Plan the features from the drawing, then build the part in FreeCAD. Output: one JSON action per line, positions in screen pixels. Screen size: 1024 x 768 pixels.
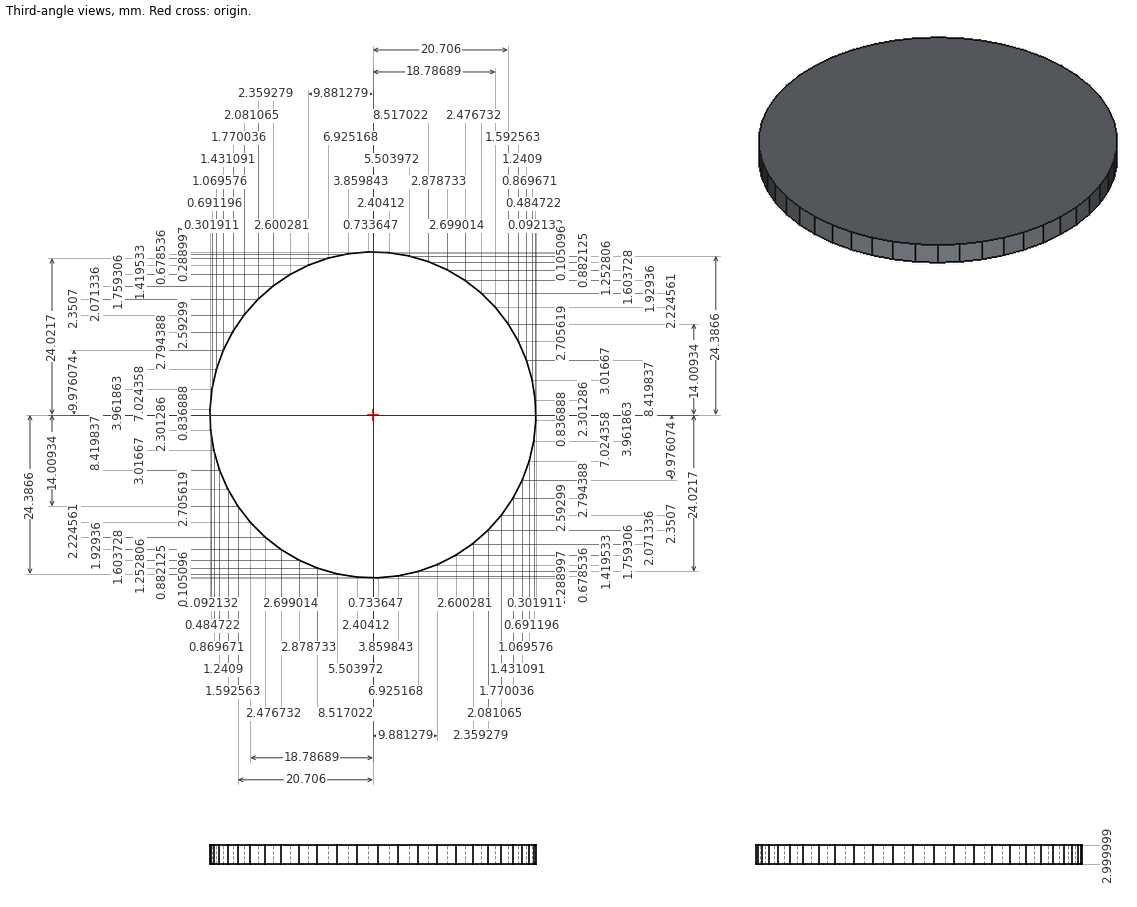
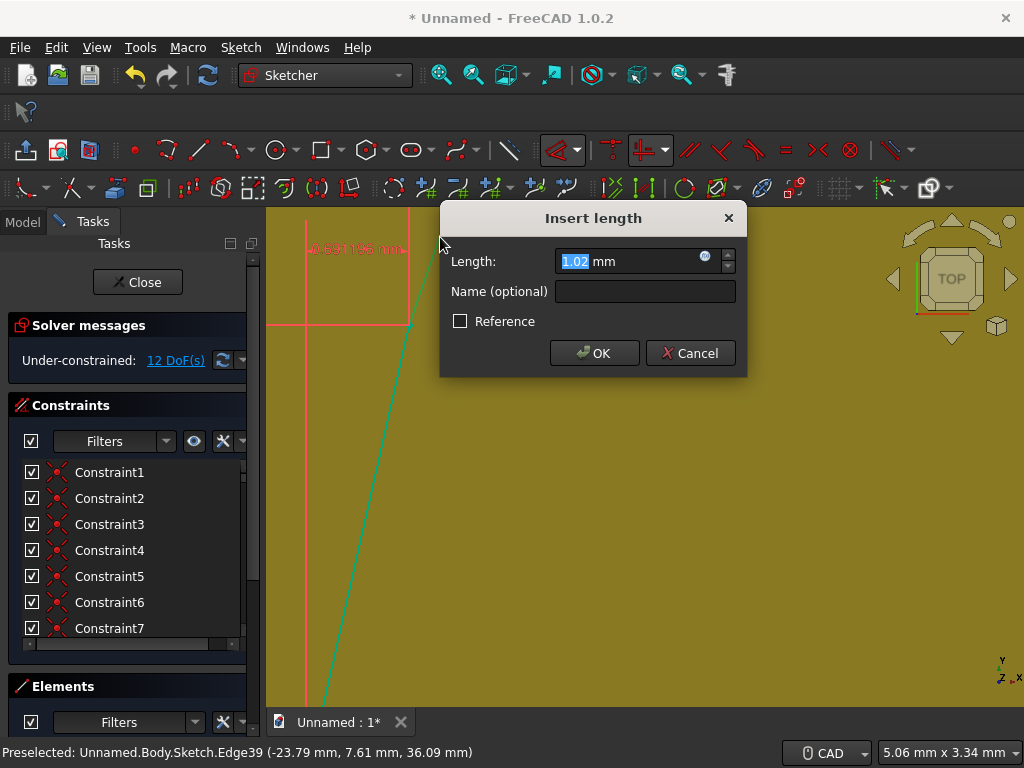
{"action": "type", "text": "1.069576"}
{"action": "key", "text": "Return"}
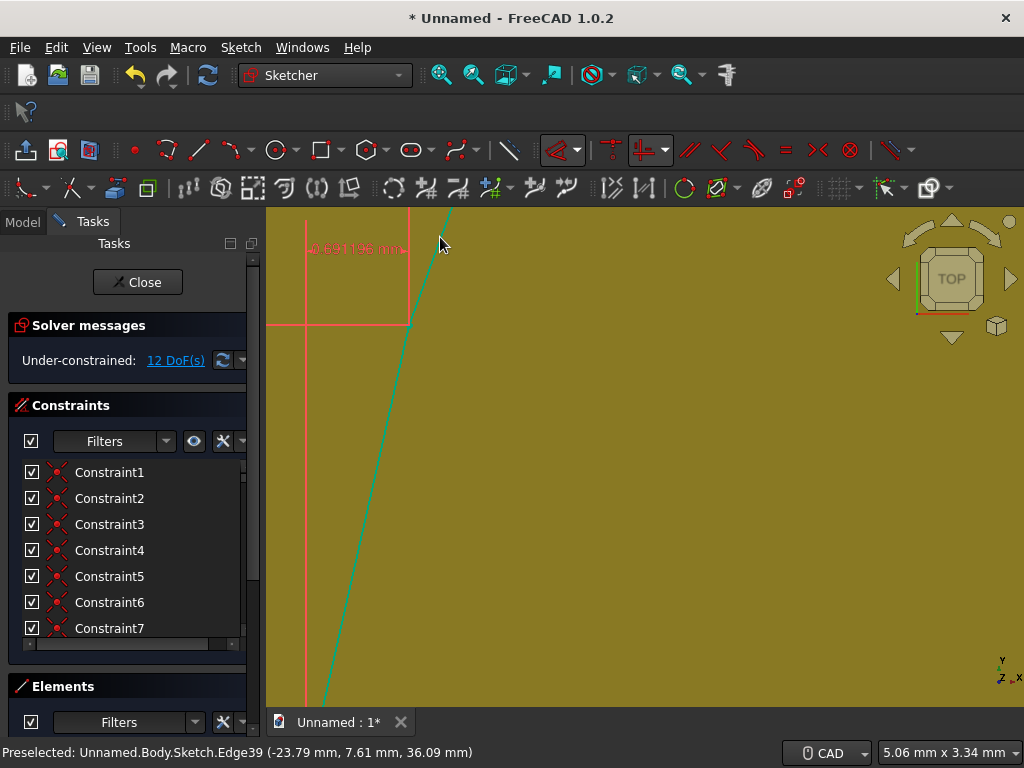
{"action": "scroll", "coordinate": [397, 409], "scroll_direction": "down", "scroll_amount": 15}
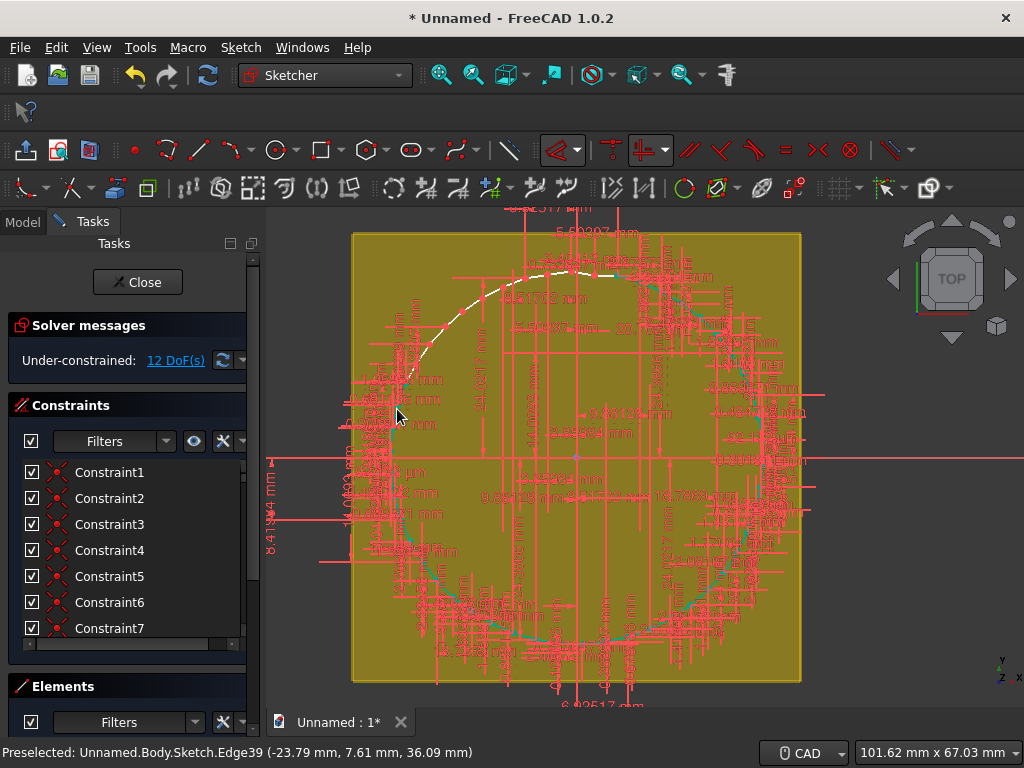
{"action": "scroll", "coordinate": [409, 377], "scroll_direction": "up", "scroll_amount": 7}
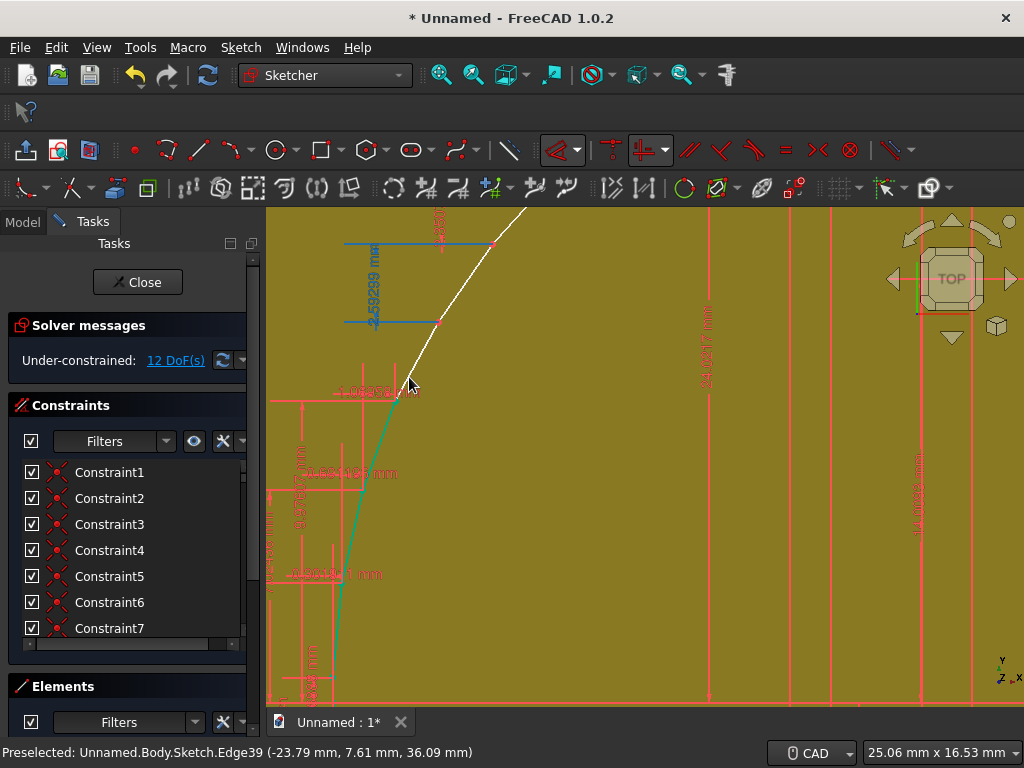
{"action": "left_click", "coordinate": [408, 378]}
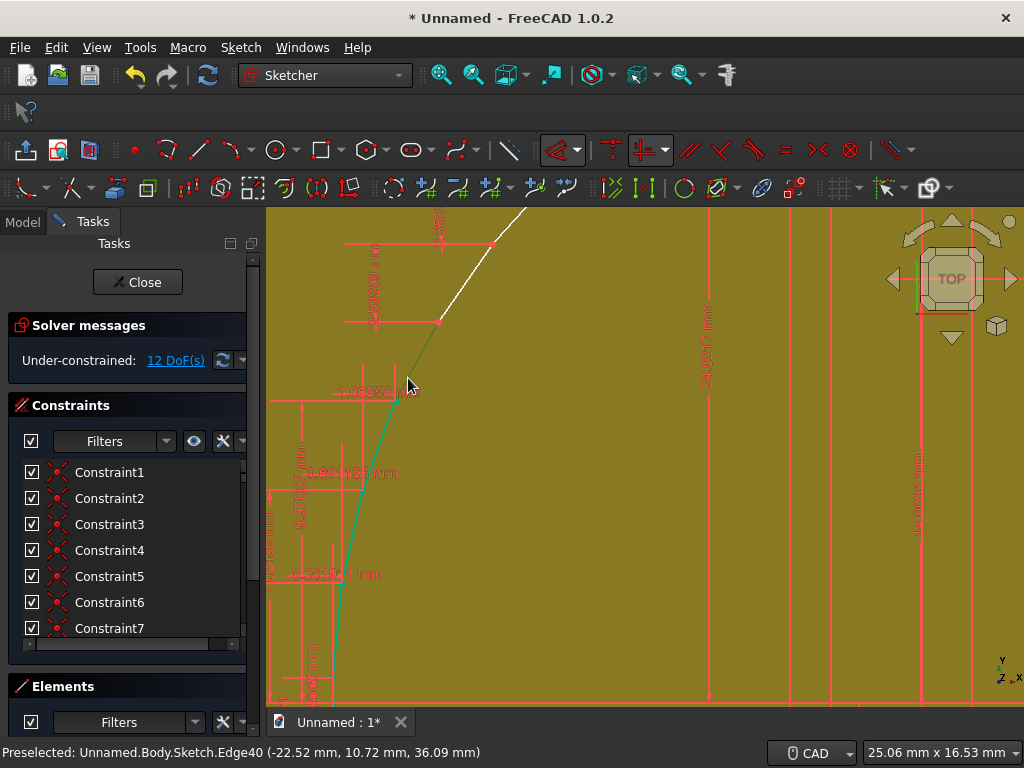
{"action": "left_click", "coordinate": [580, 150]}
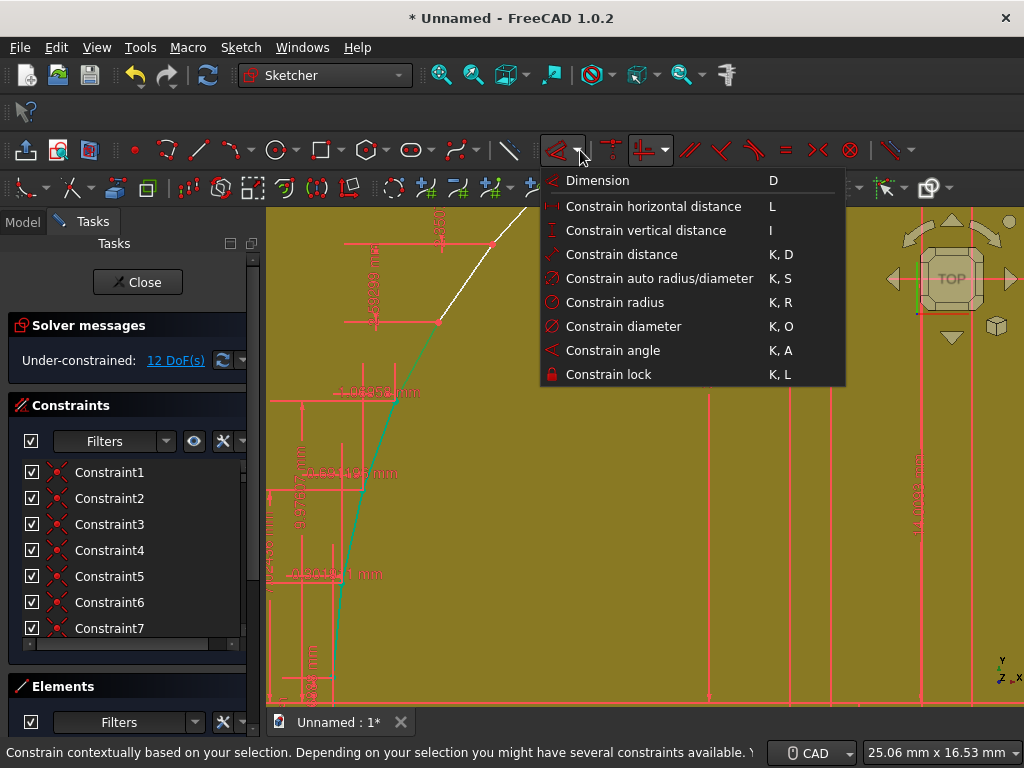
{"action": "left_click", "coordinate": [693, 206]}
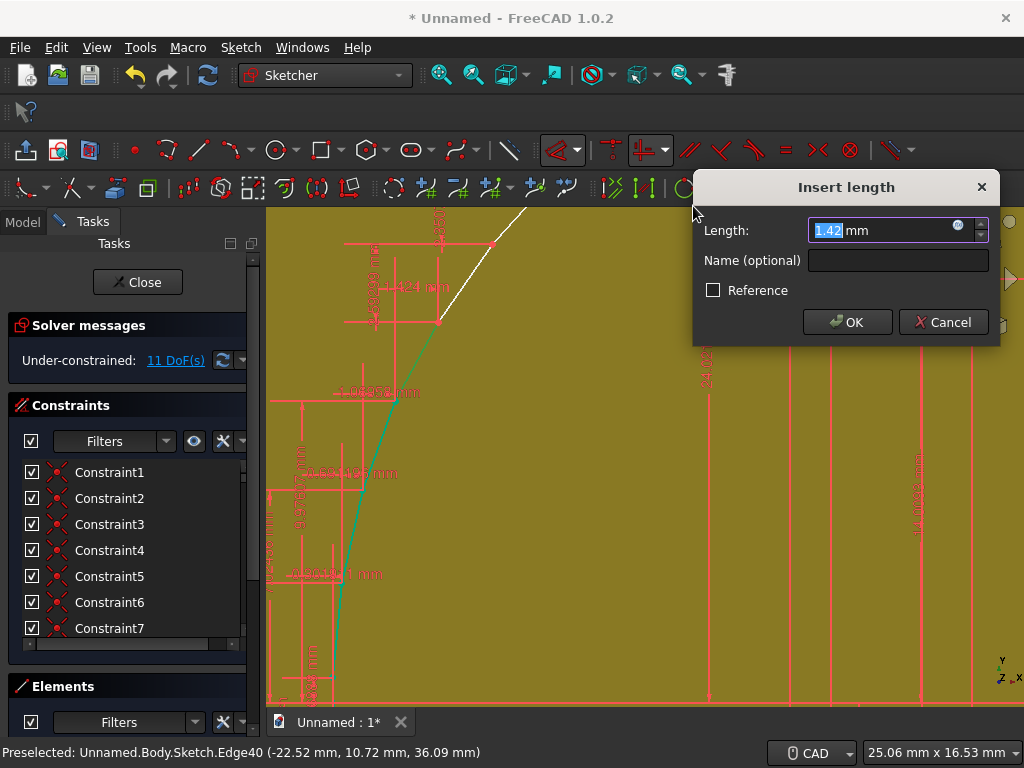
{"action": "type", "text": "1.431091"}
{"action": "key", "text": "Return"}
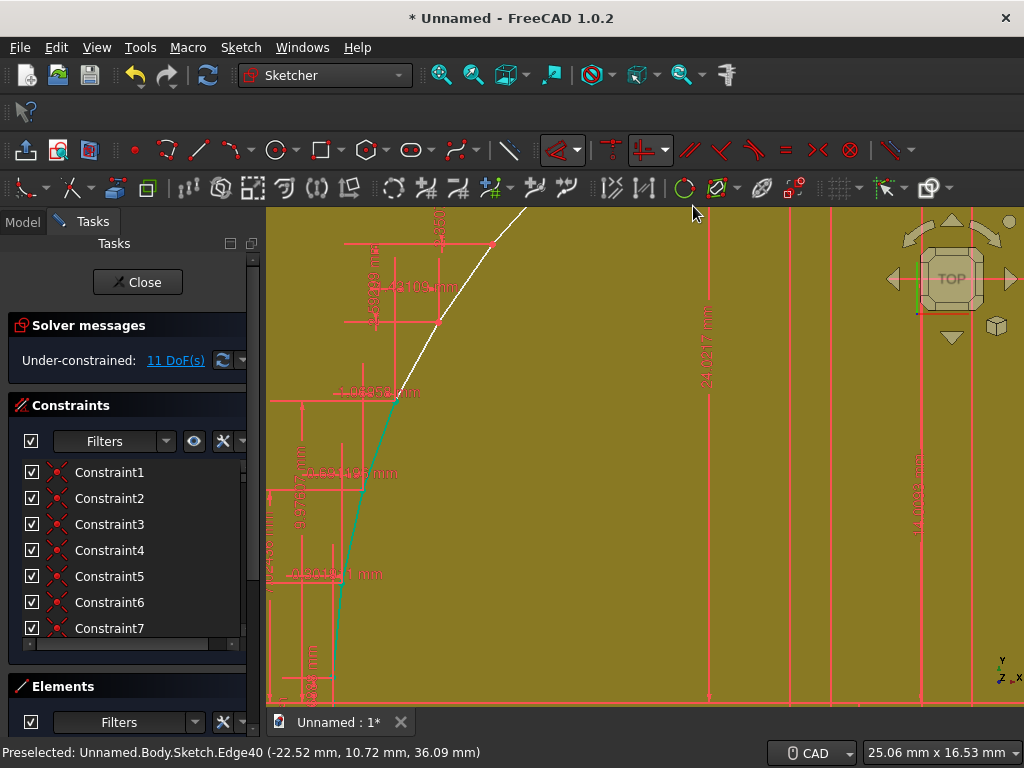
{"action": "left_click", "coordinate": [408, 378]}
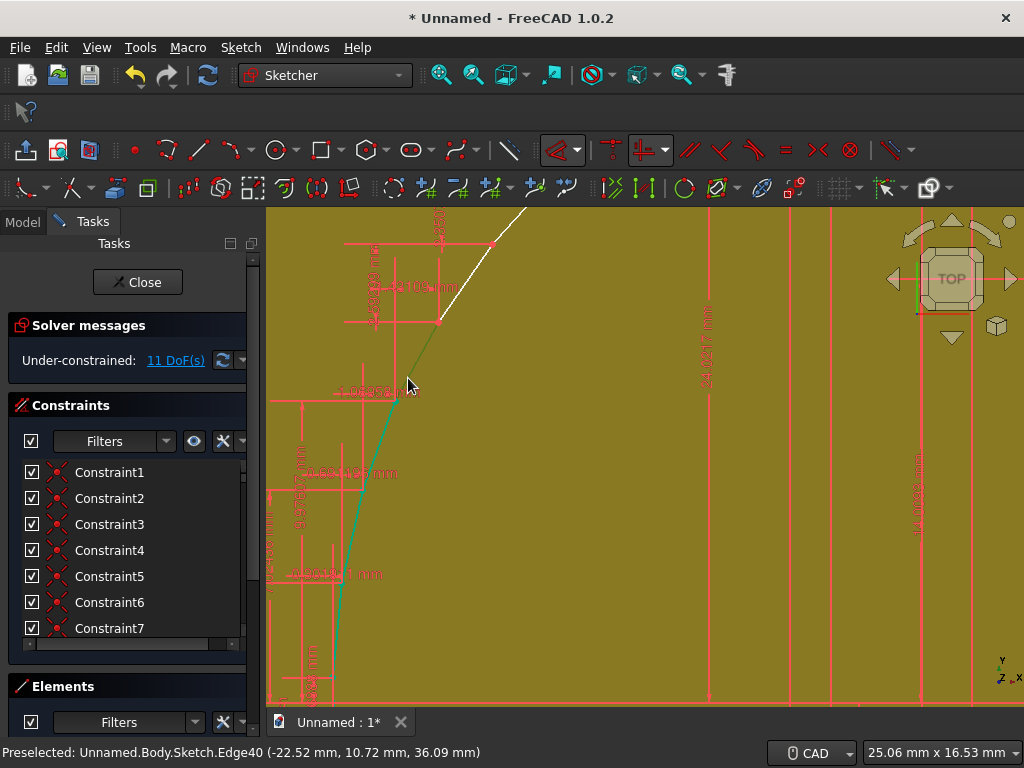
{"action": "left_click", "coordinate": [580, 150]}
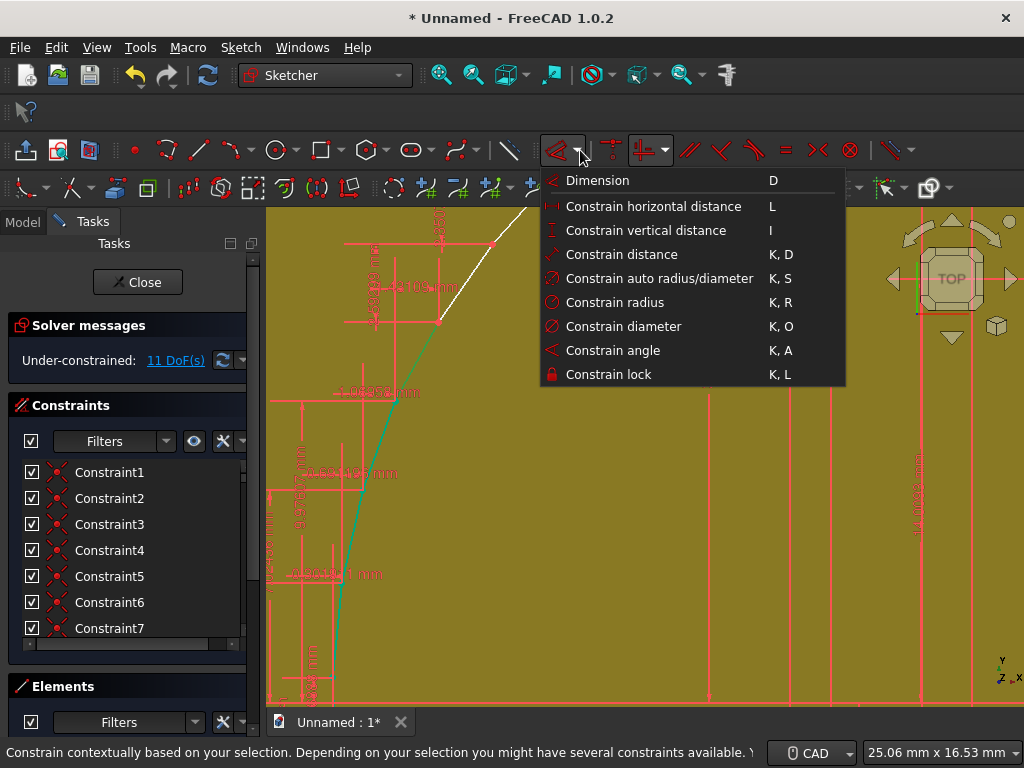
{"action": "left_click", "coordinate": [693, 230]}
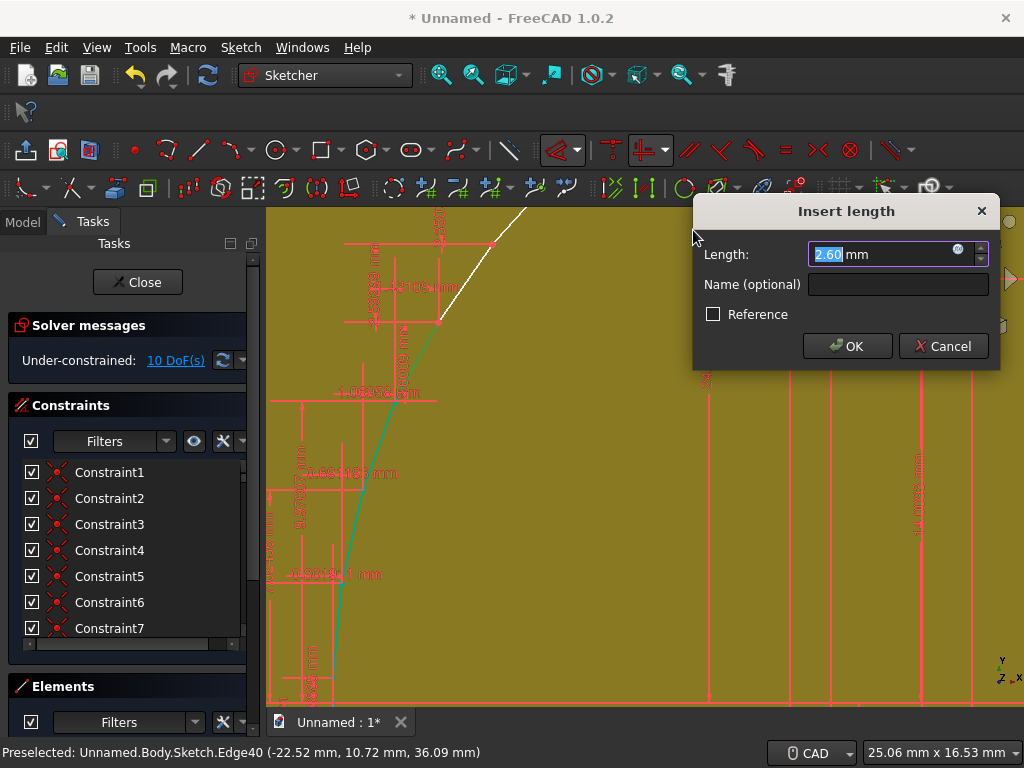
{"action": "type", "text": "2.794388"}
{"action": "key", "text": "Return"}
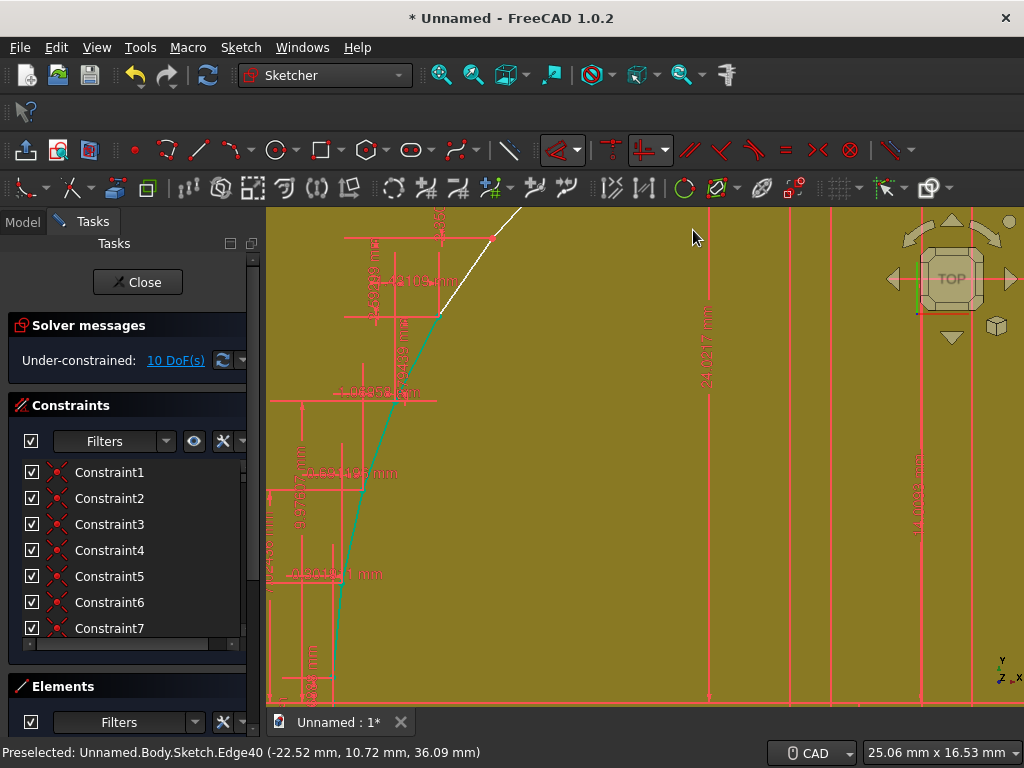
{"action": "left_click", "coordinate": [455, 293]}